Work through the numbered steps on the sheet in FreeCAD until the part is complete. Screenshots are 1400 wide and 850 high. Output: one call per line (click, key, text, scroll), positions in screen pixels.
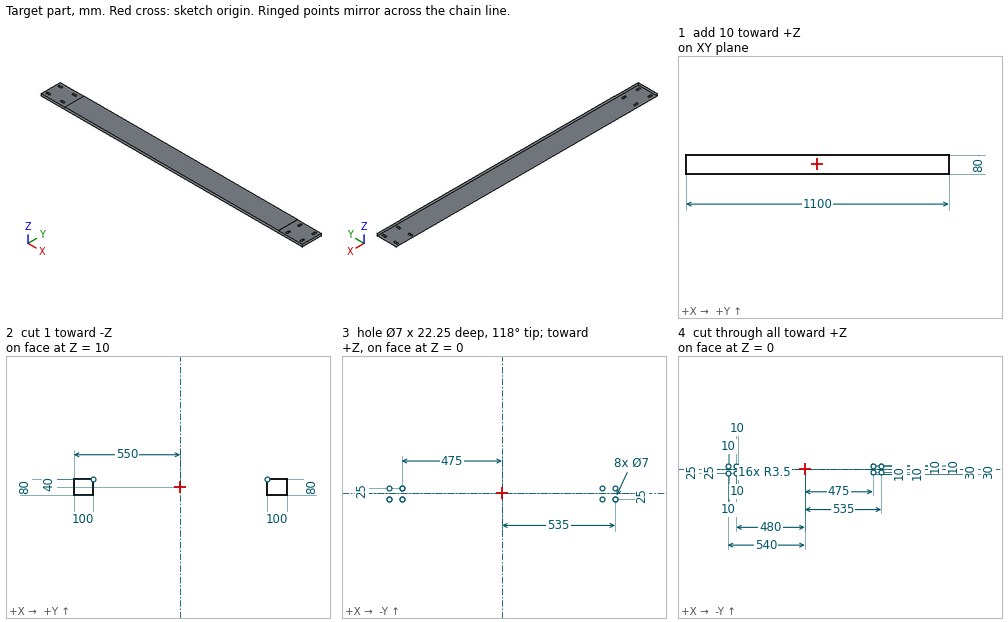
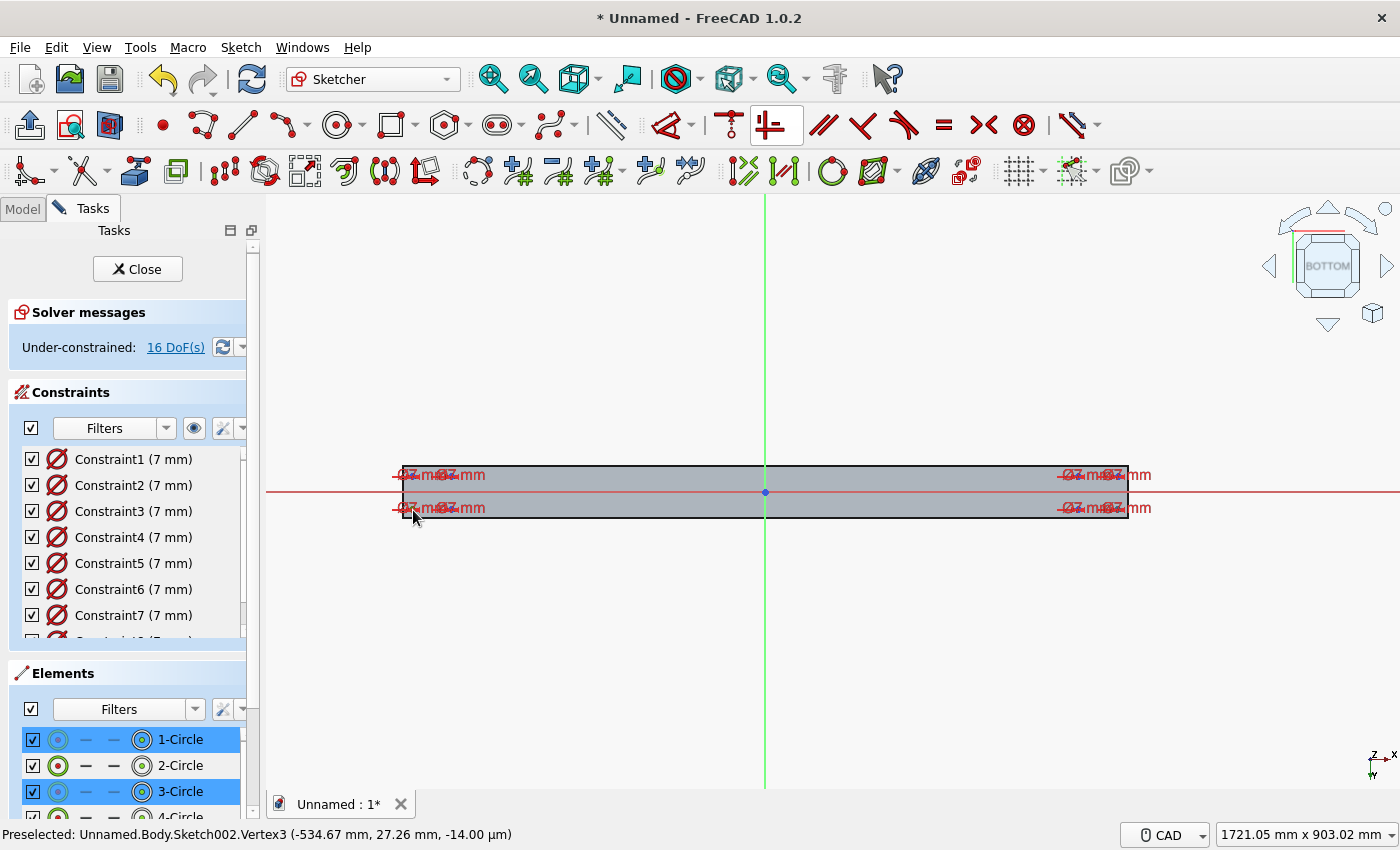
click(765, 722)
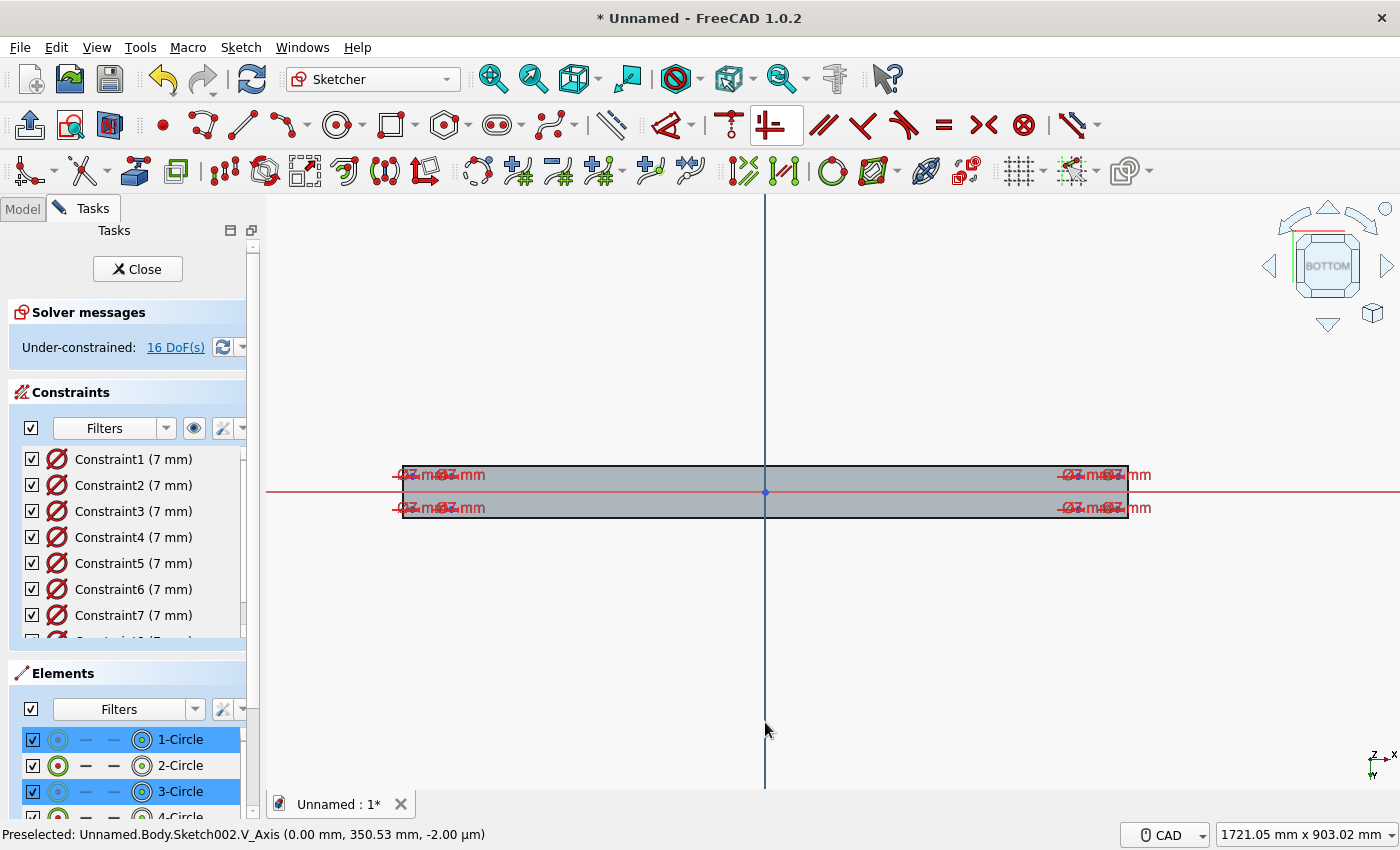
key(s)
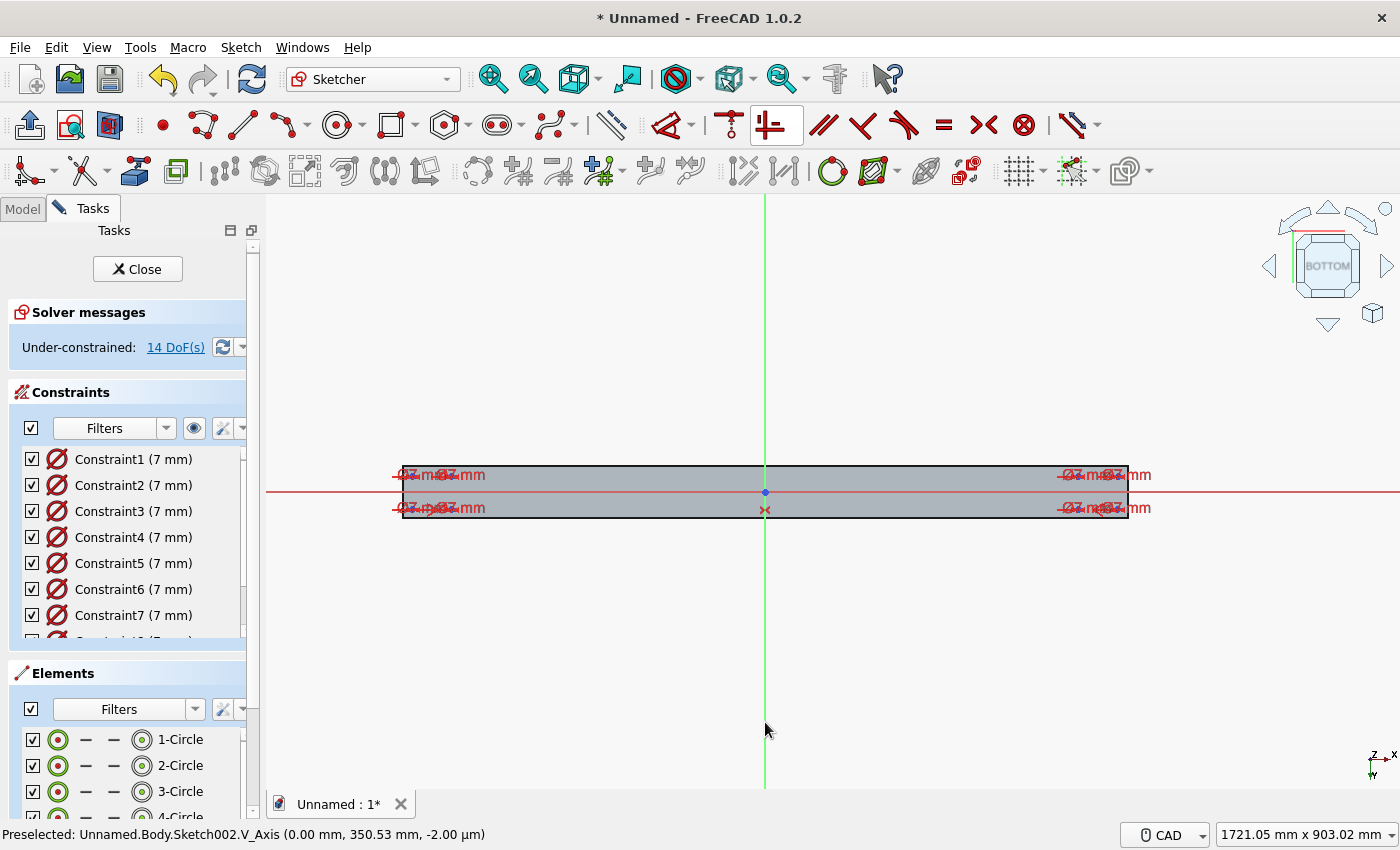
click(413, 510)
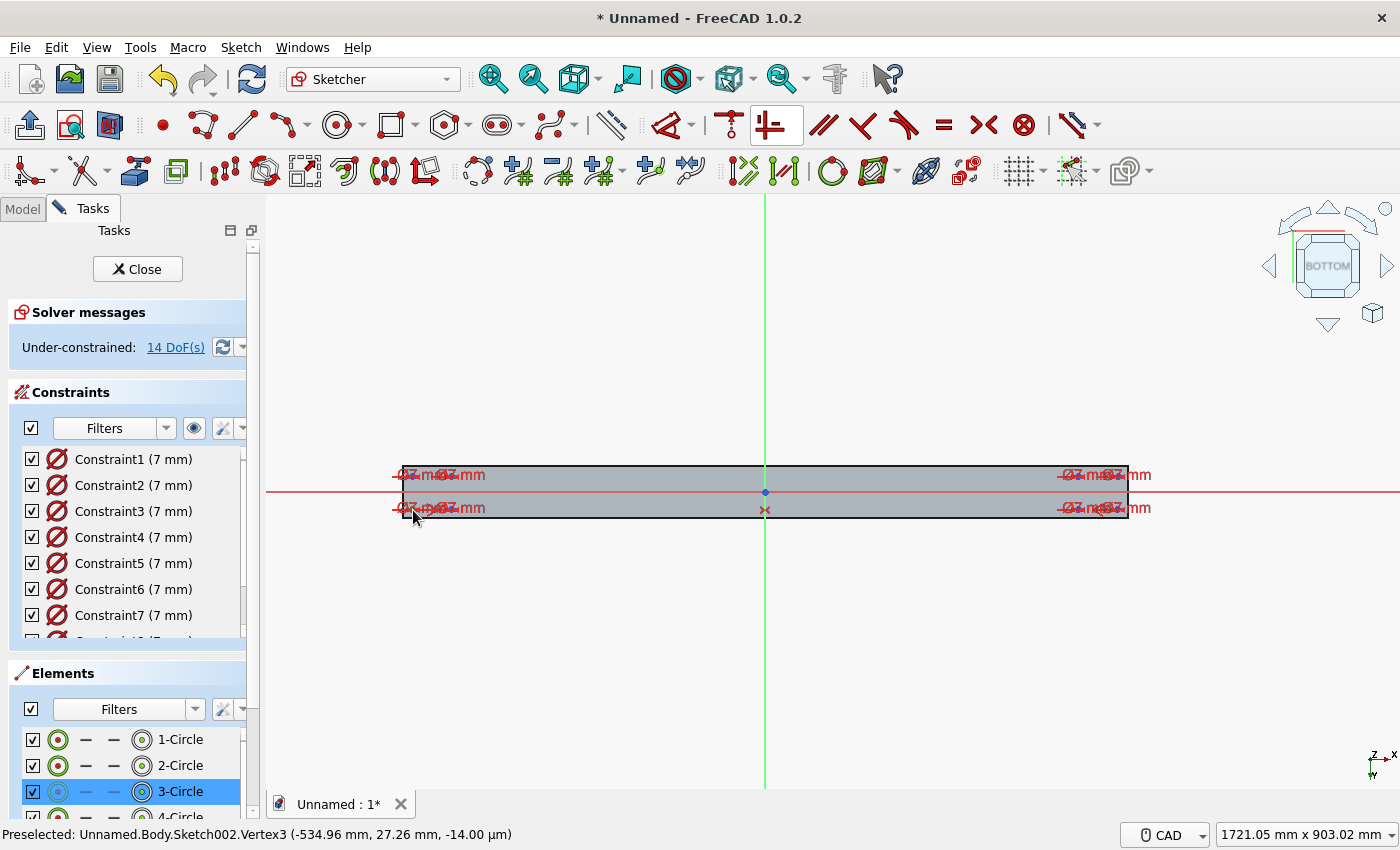
click(413, 477)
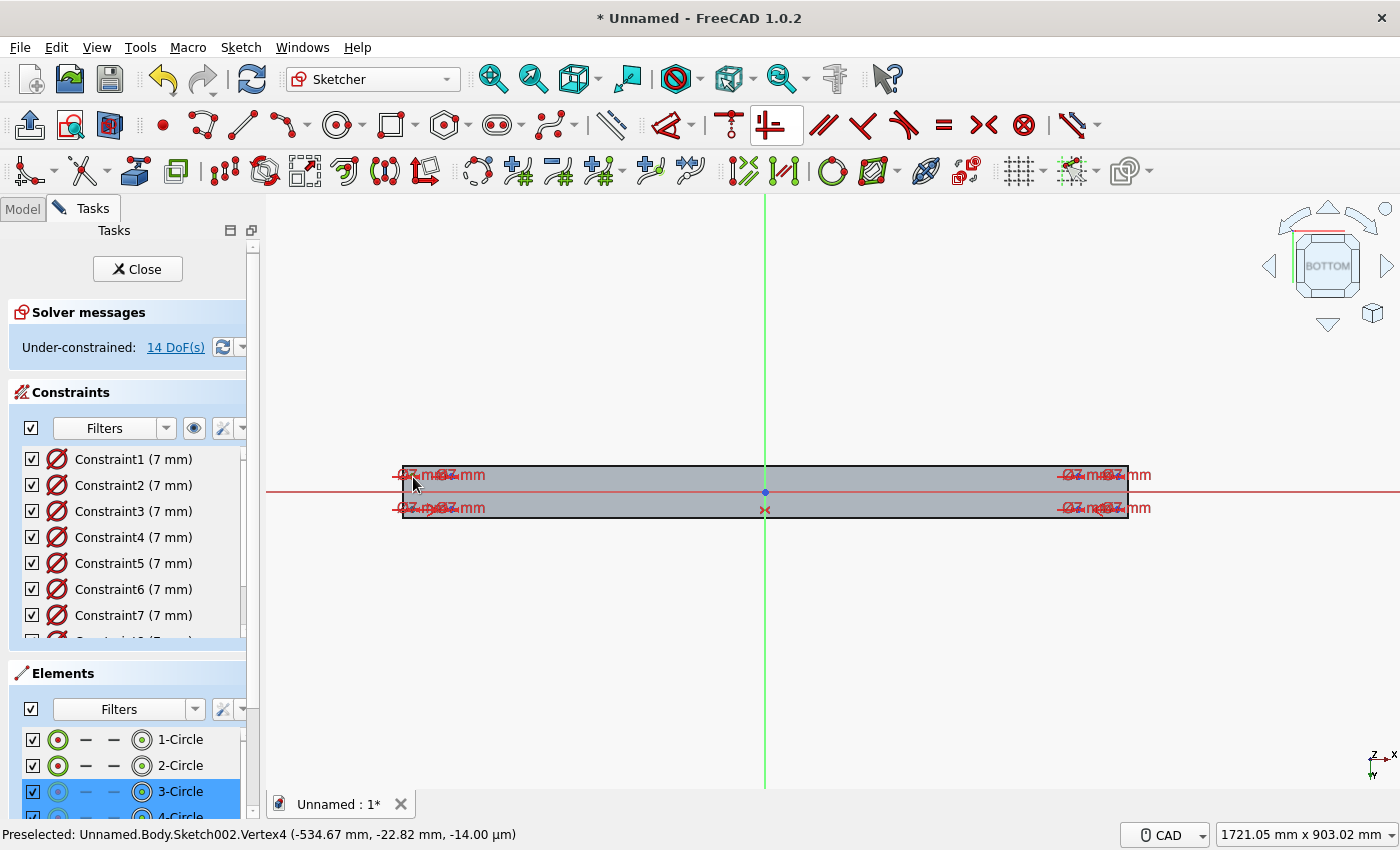
click(361, 492)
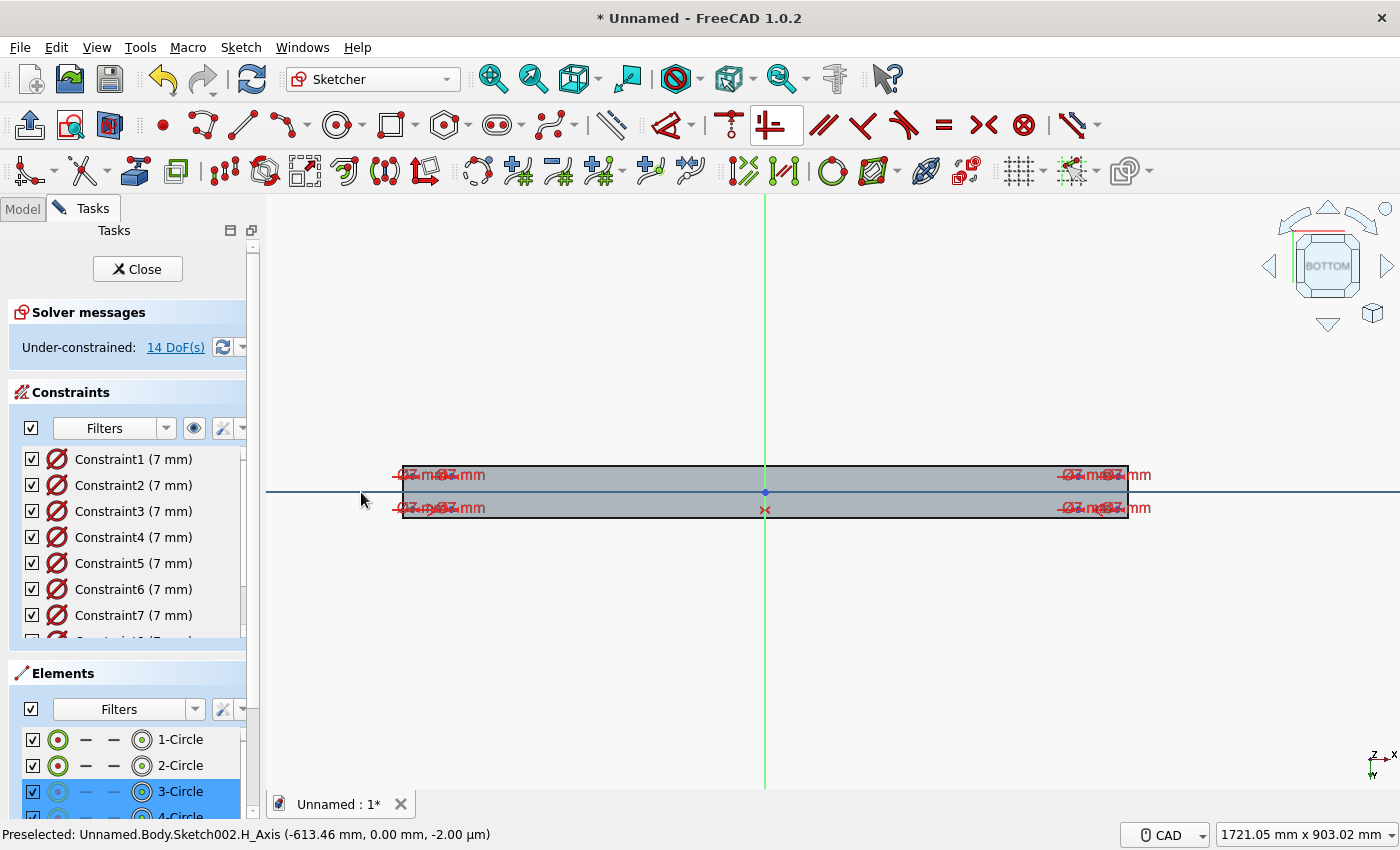
key(s)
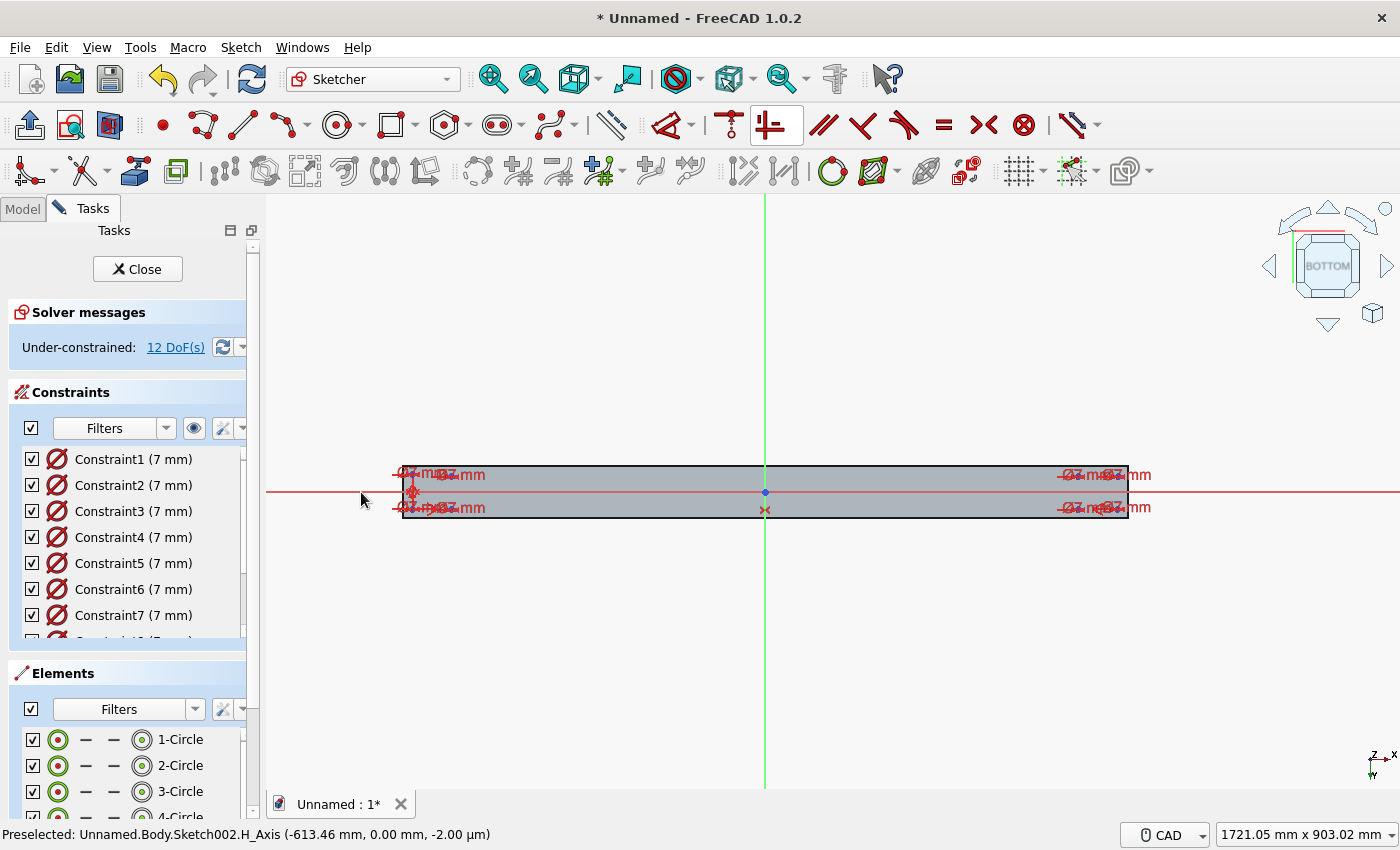
click(452, 477)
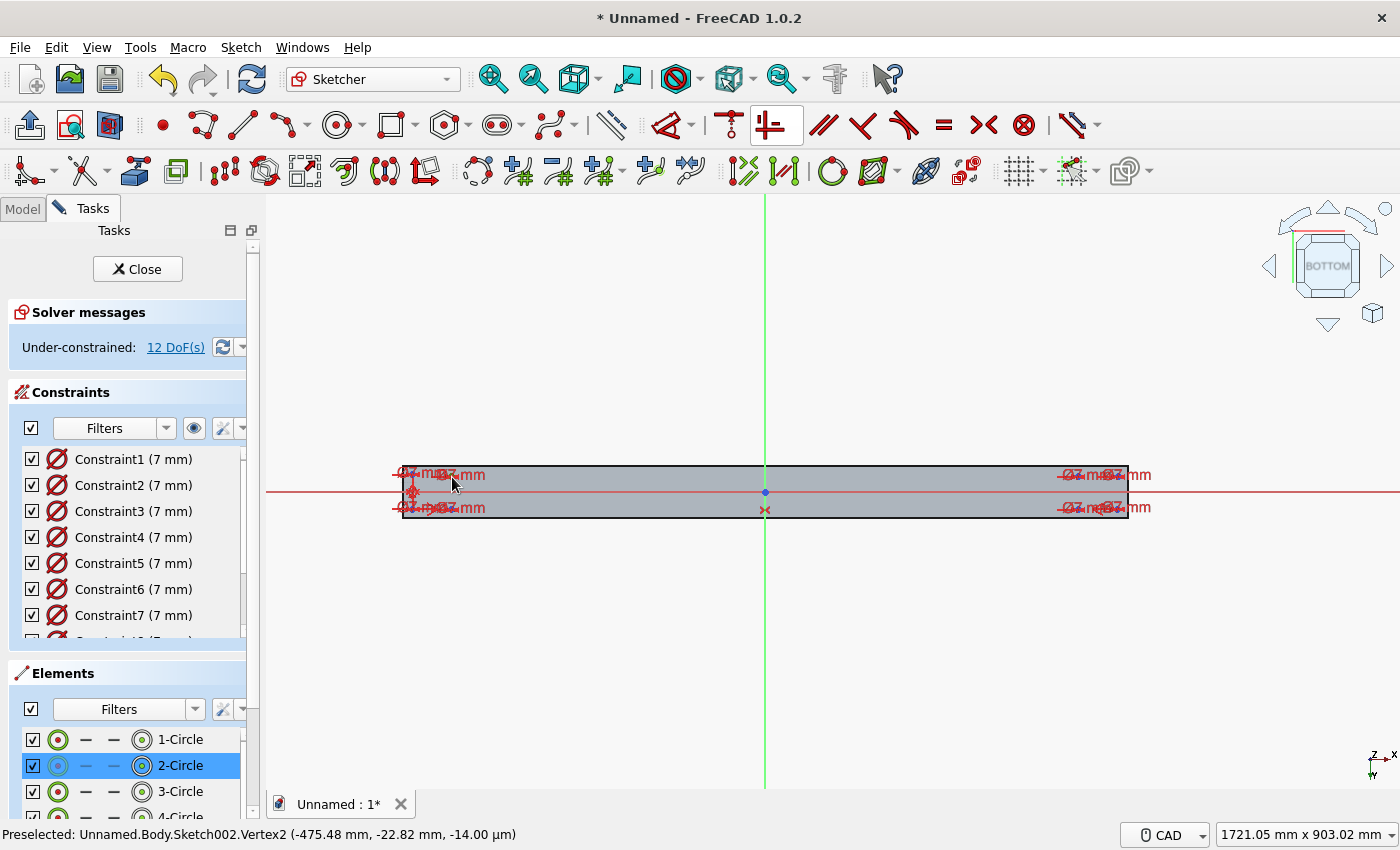
click(452, 510)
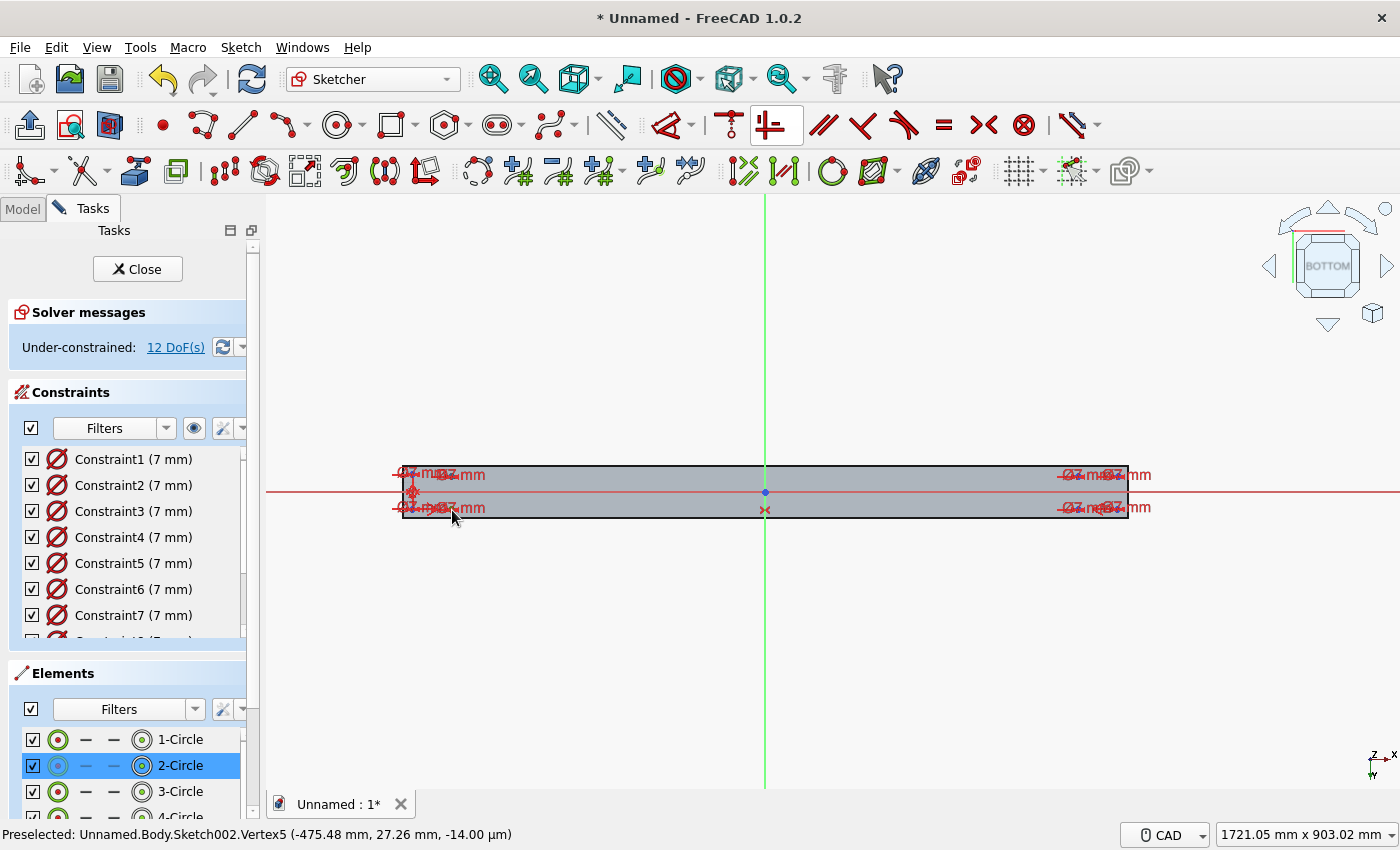
click(361, 492)